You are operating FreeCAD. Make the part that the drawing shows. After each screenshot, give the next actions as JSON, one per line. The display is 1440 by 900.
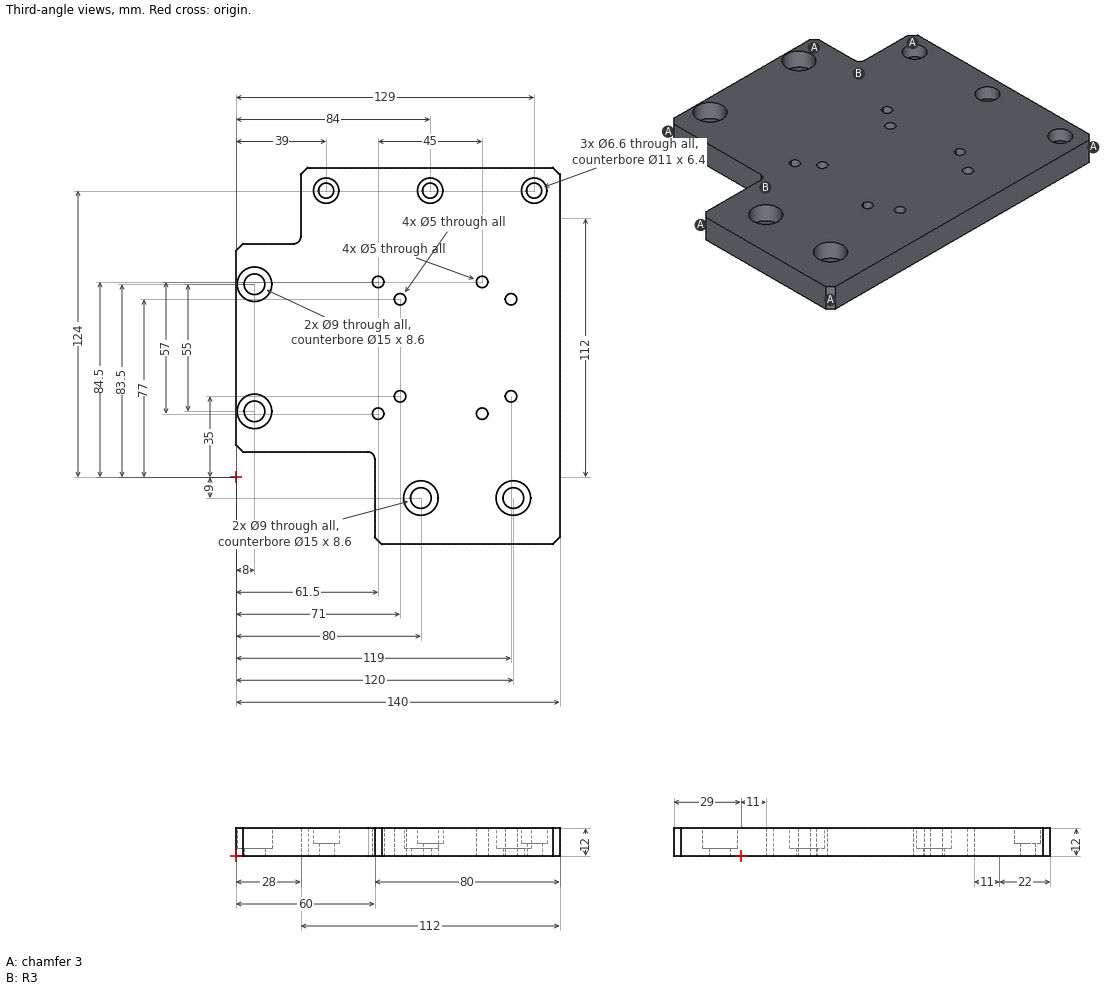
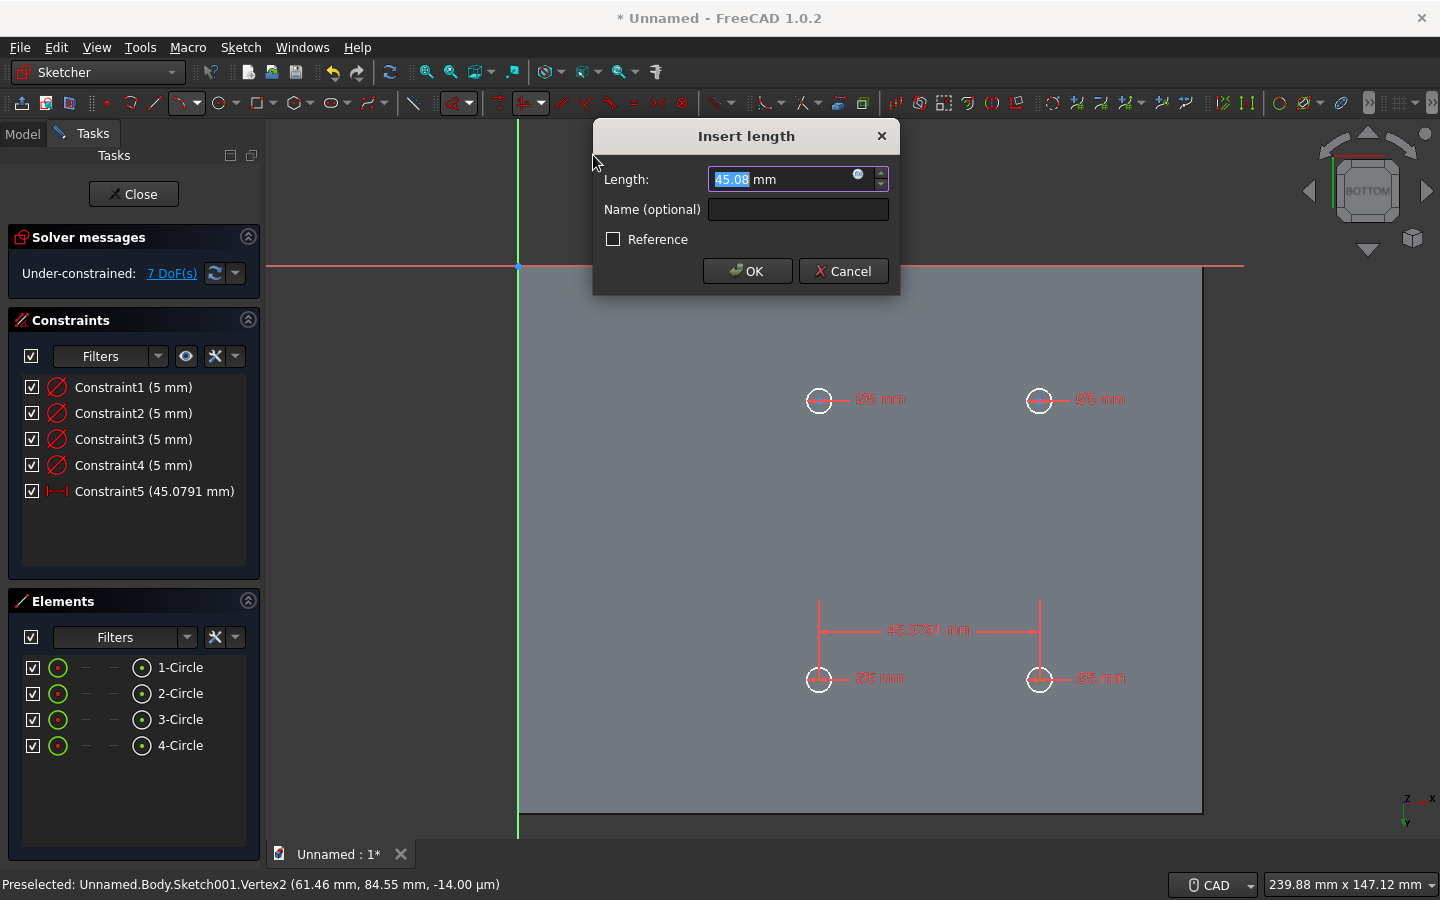
{"action": "type", "text": "45"}
{"action": "key", "text": "Return"}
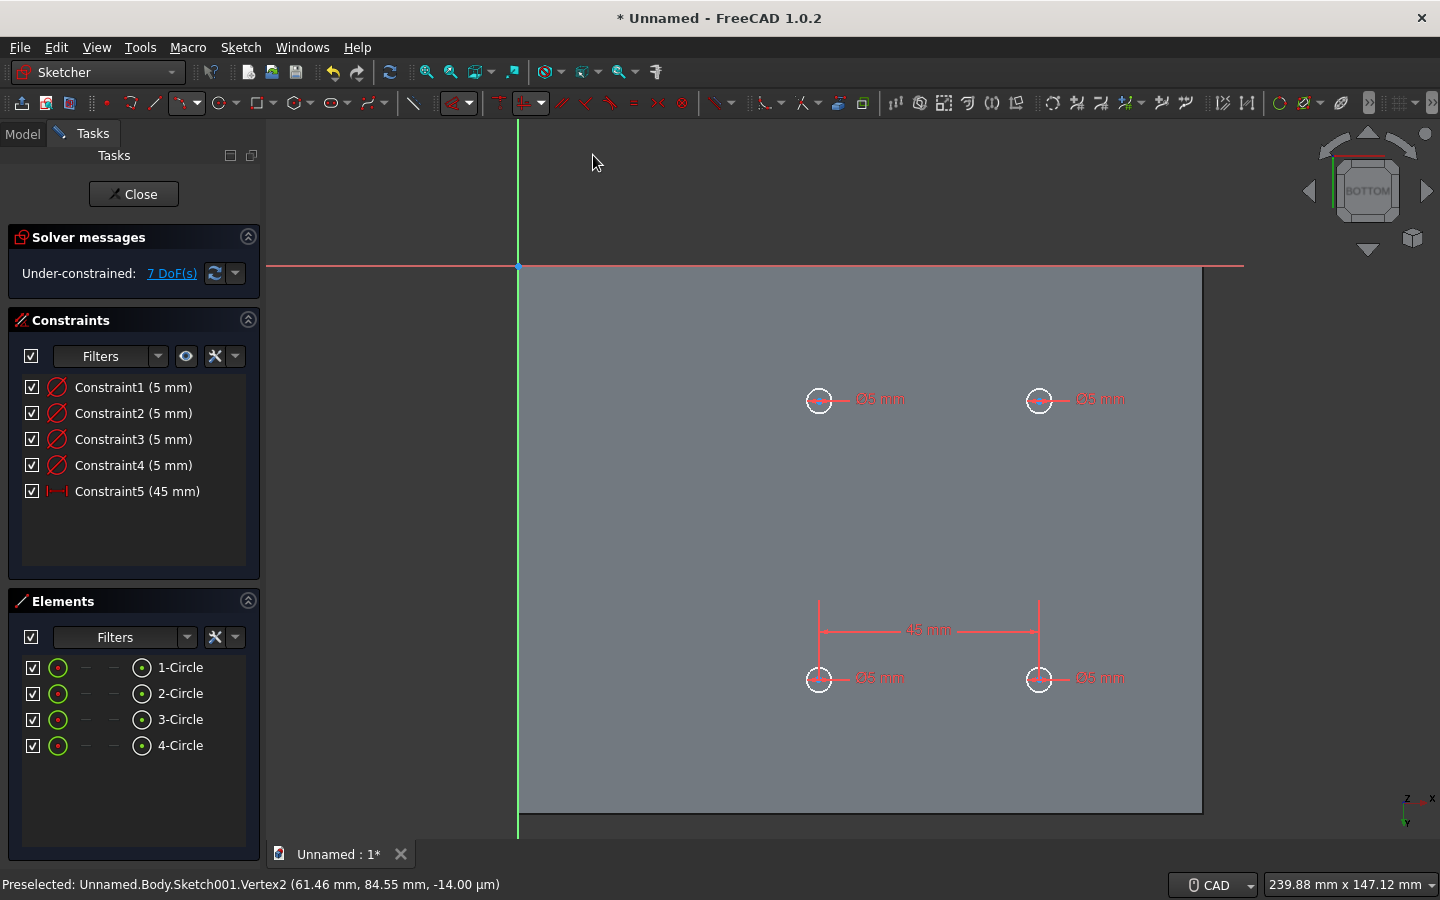
{"action": "left_click", "coordinate": [1039, 680]}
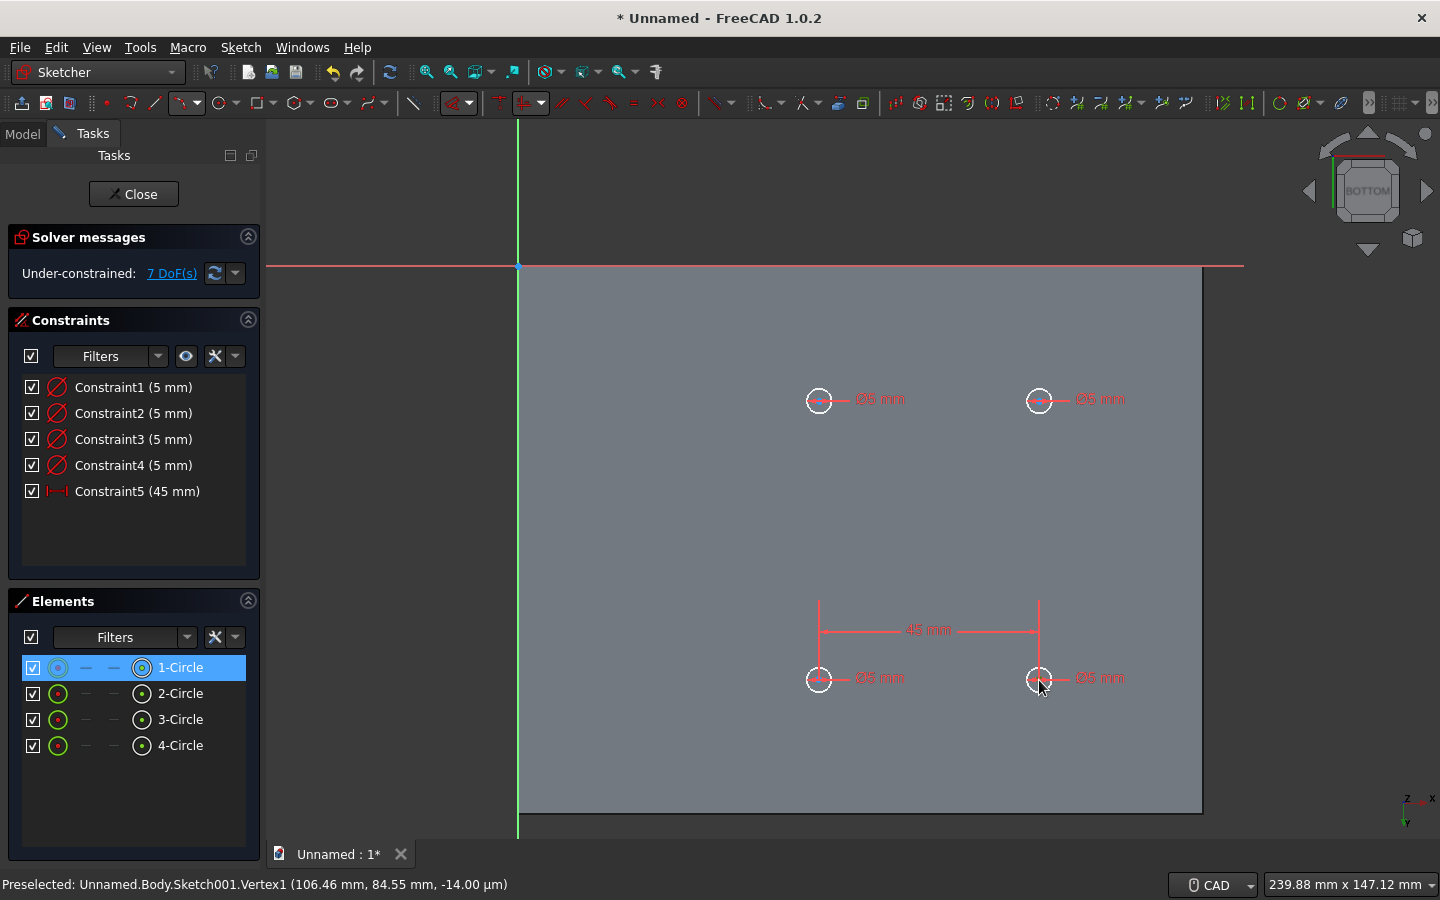
{"action": "left_click", "coordinate": [819, 401]}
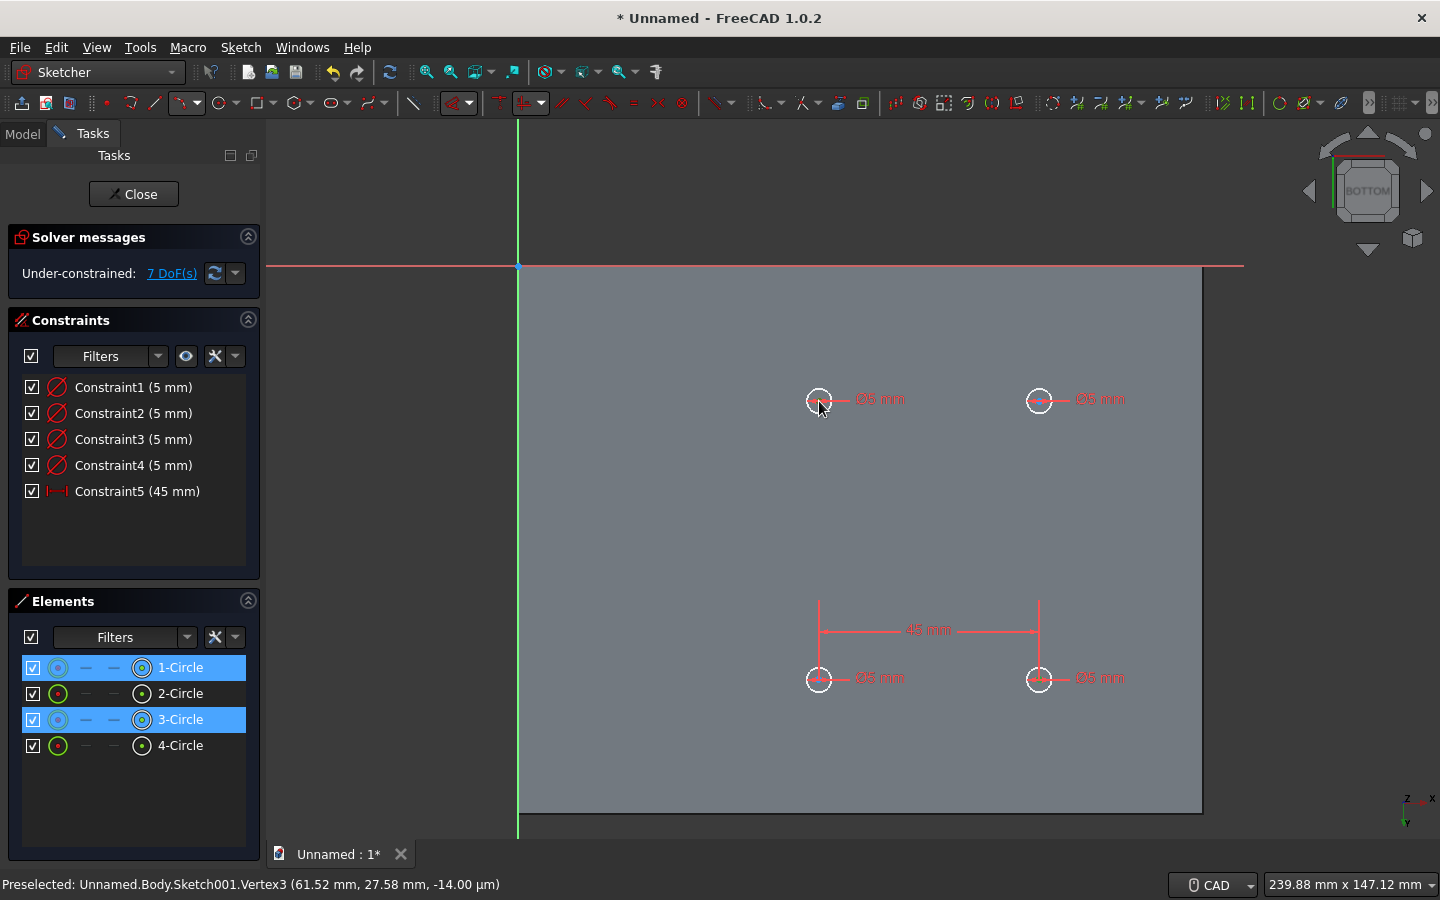
{"action": "left_click", "coordinate": [472, 104]}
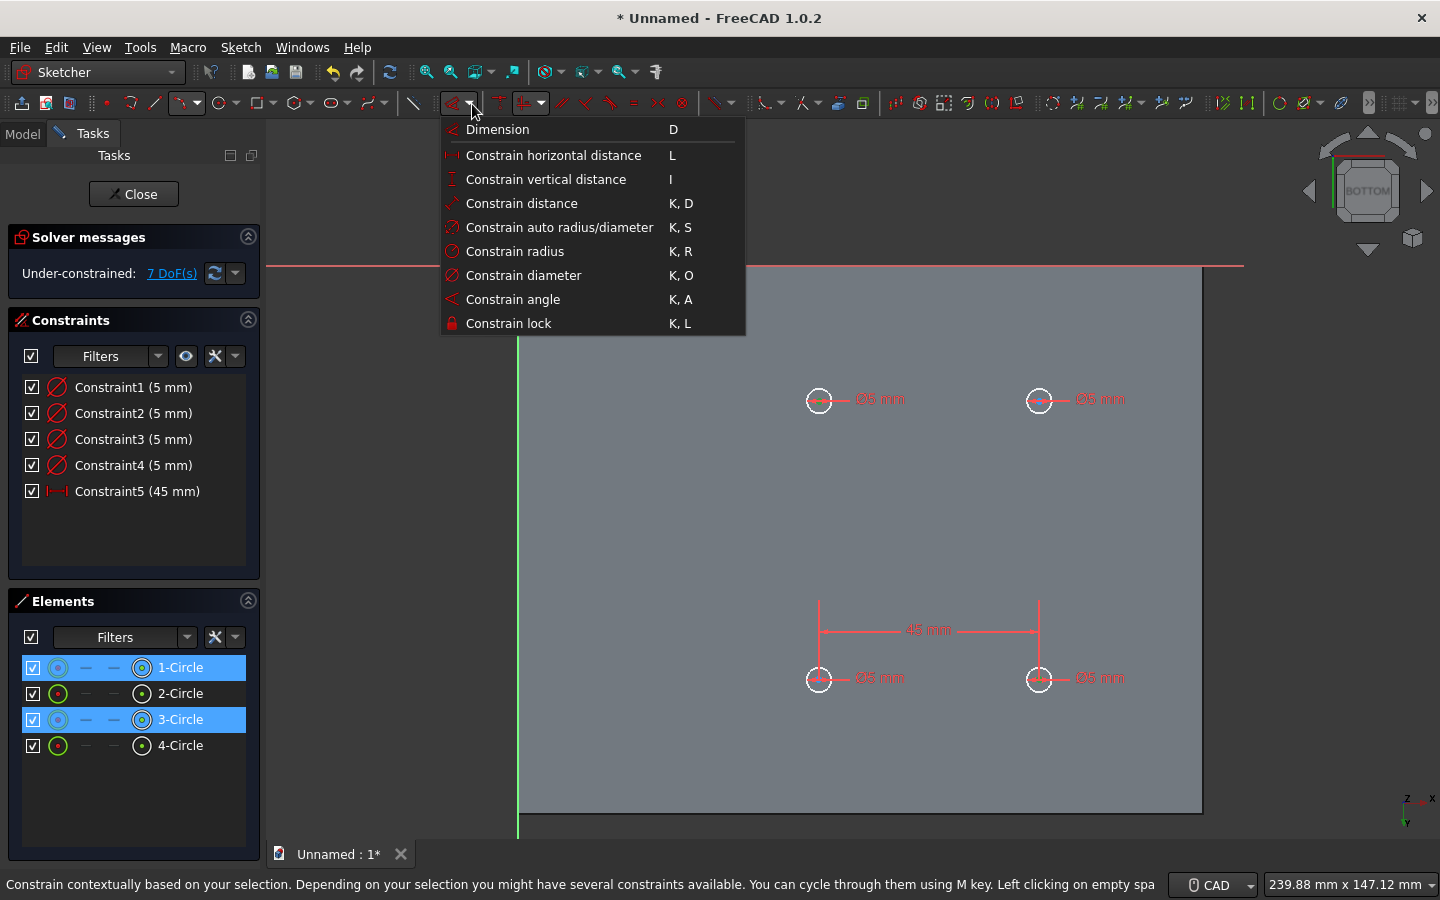
{"action": "left_click", "coordinate": [593, 155]}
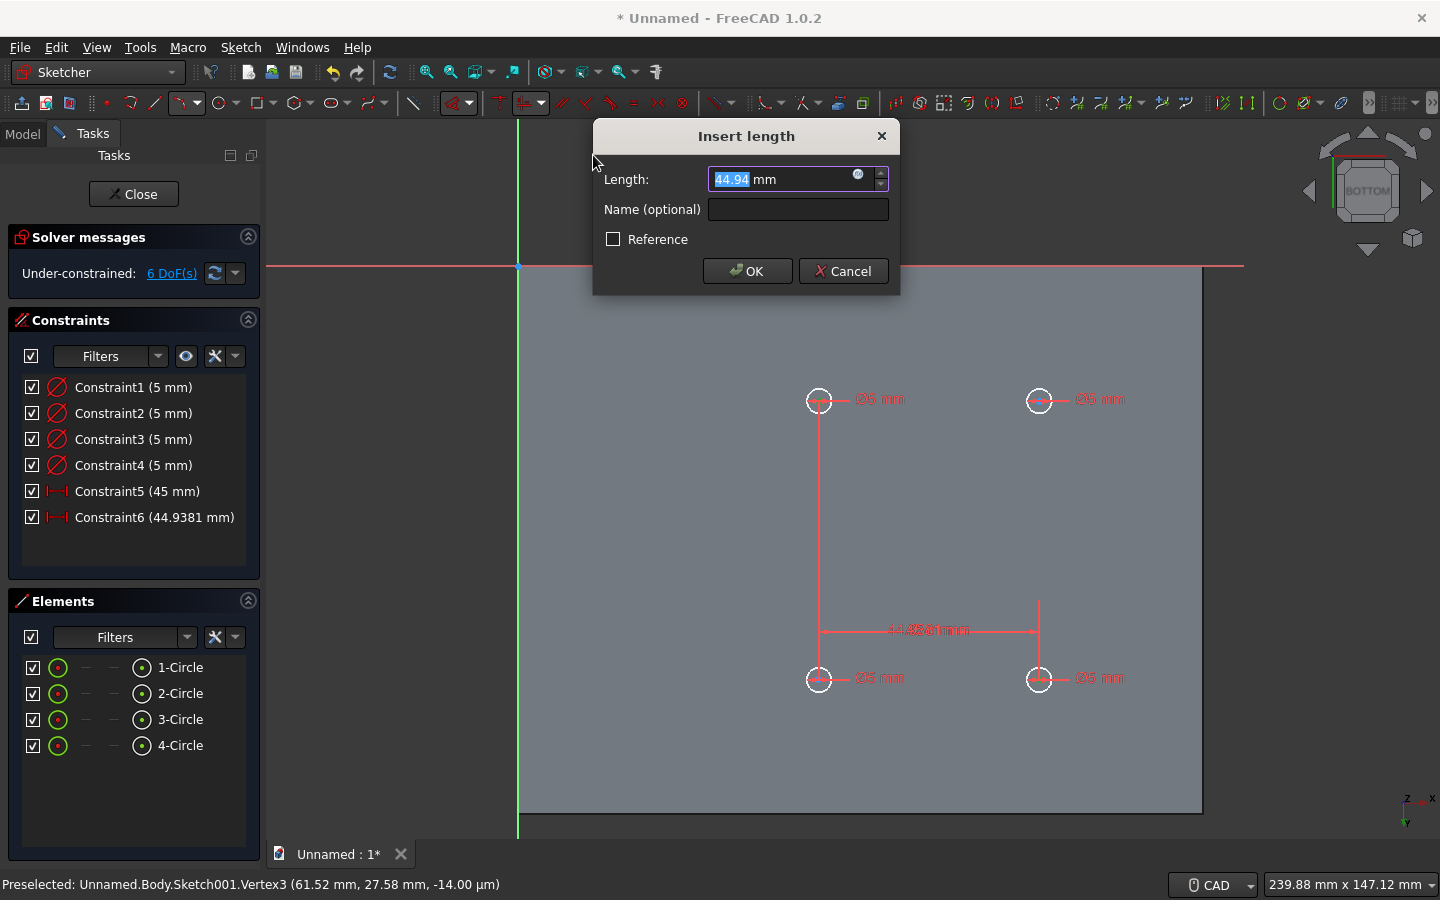
{"action": "type", "text": "45"}
{"action": "key", "text": "Return"}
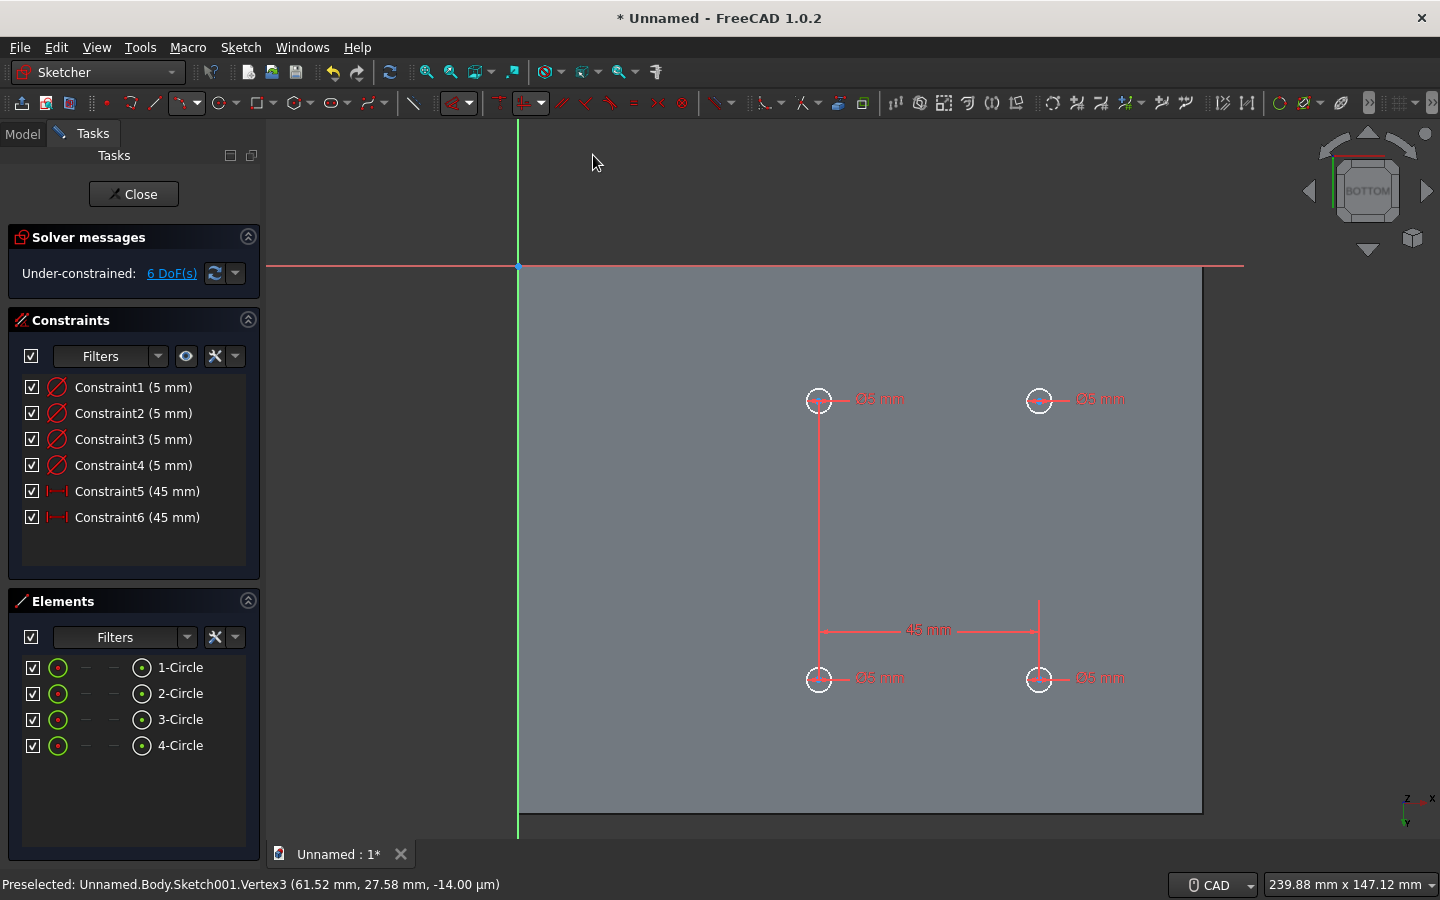
{"action": "left_click", "coordinate": [819, 680]}